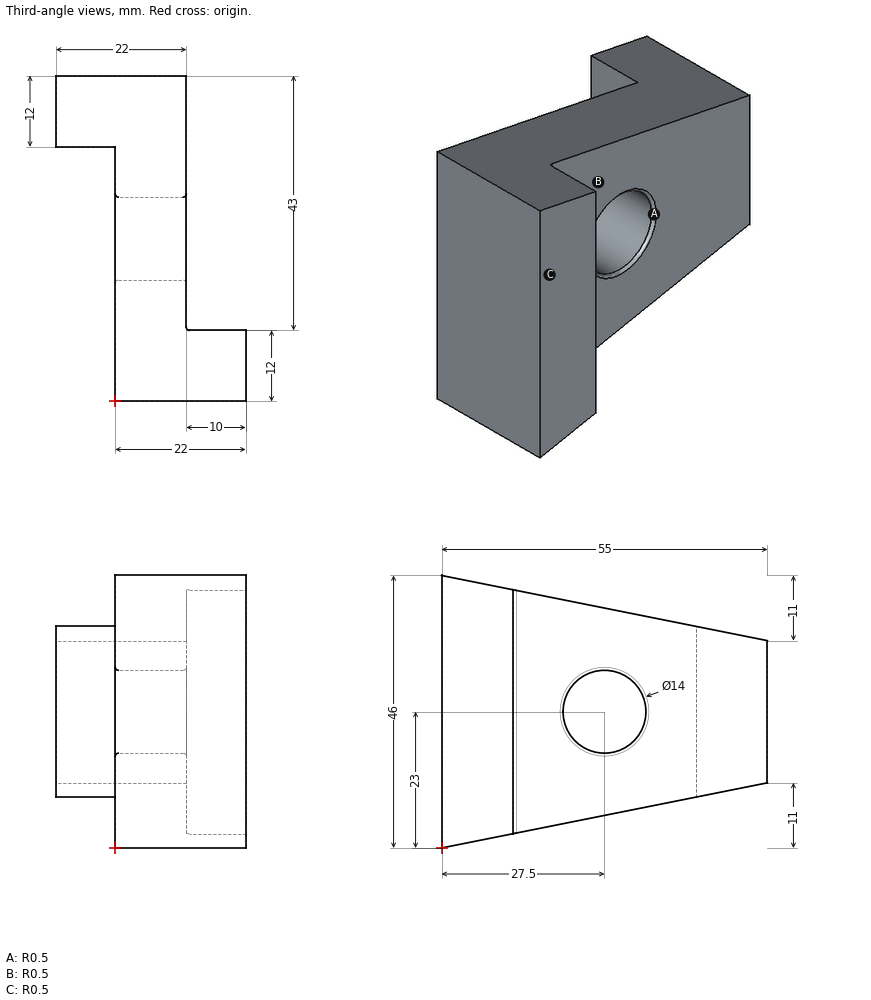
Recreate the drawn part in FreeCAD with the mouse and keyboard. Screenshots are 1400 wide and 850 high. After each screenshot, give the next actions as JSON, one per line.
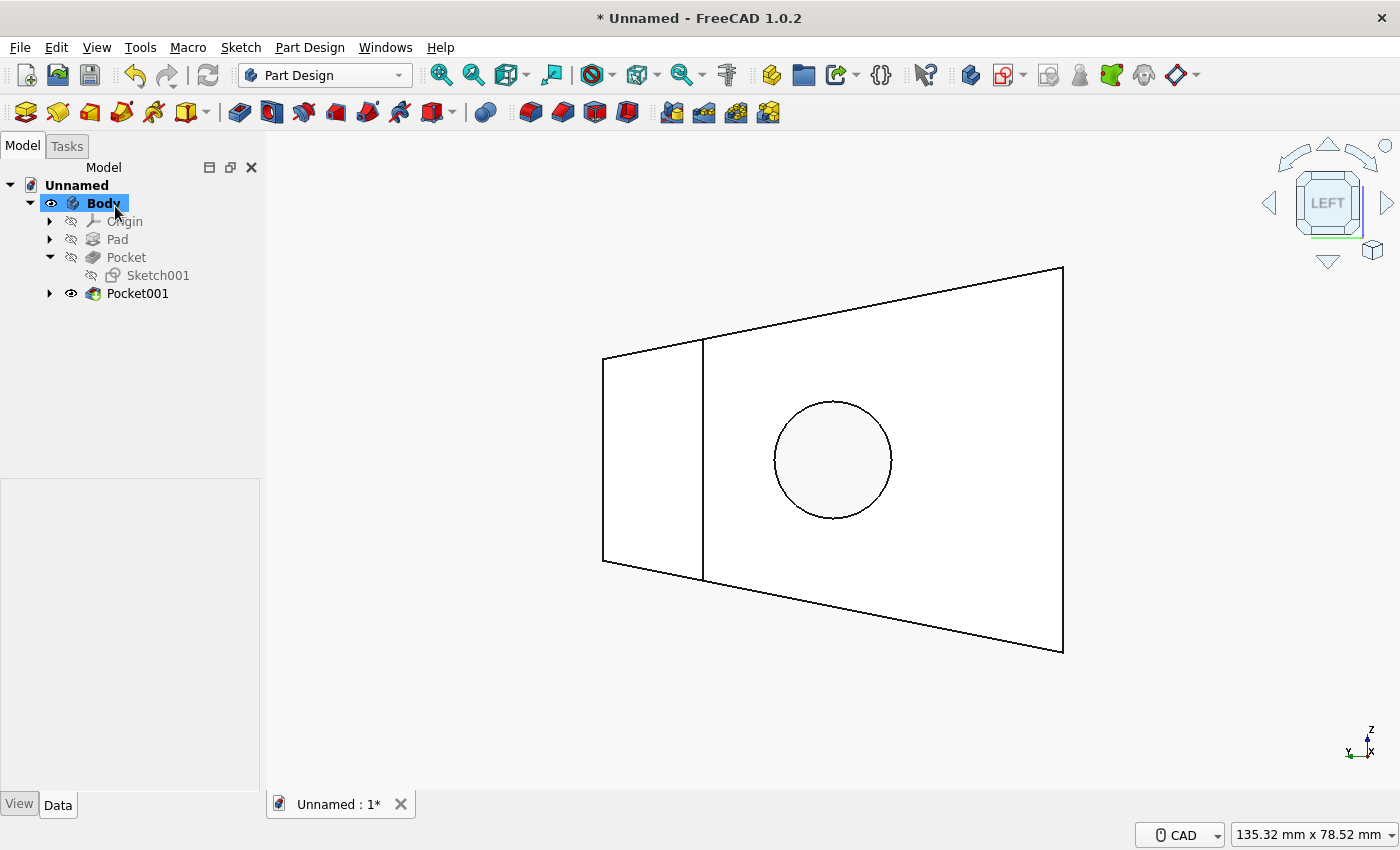
{"action": "key", "text": "0"}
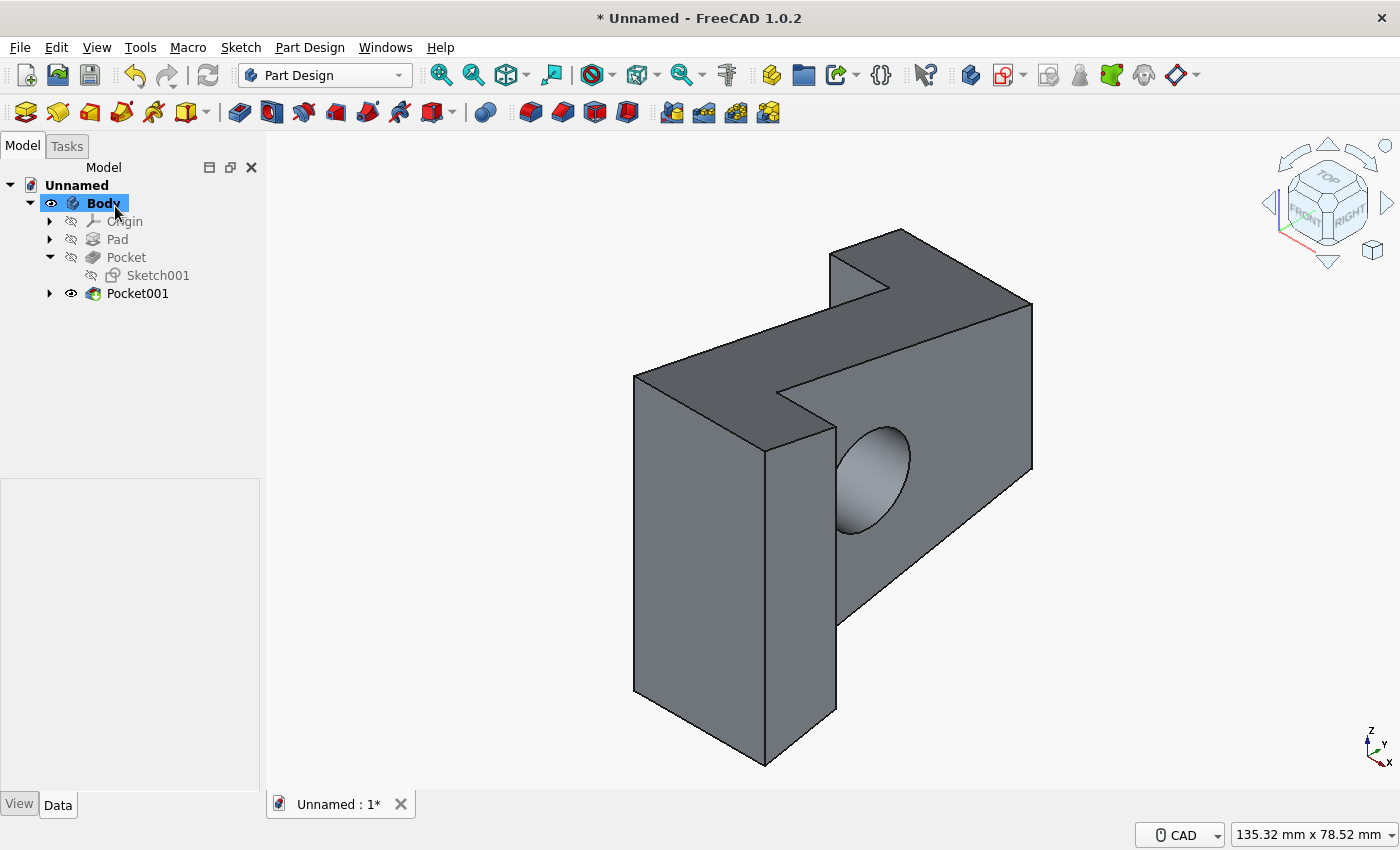
{"action": "left_click", "coordinate": [910, 456]}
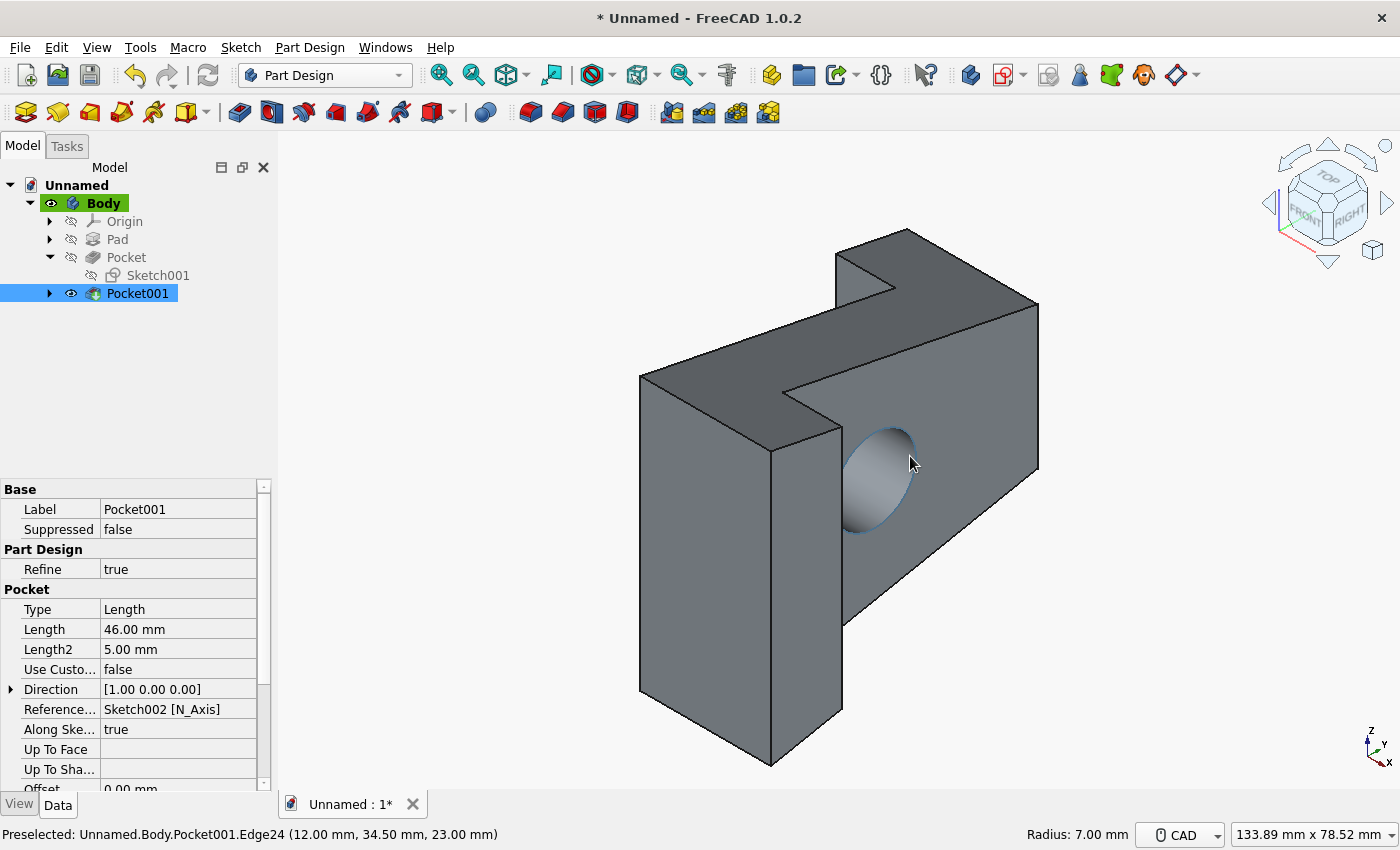
{"action": "left_click", "coordinate": [532, 112]}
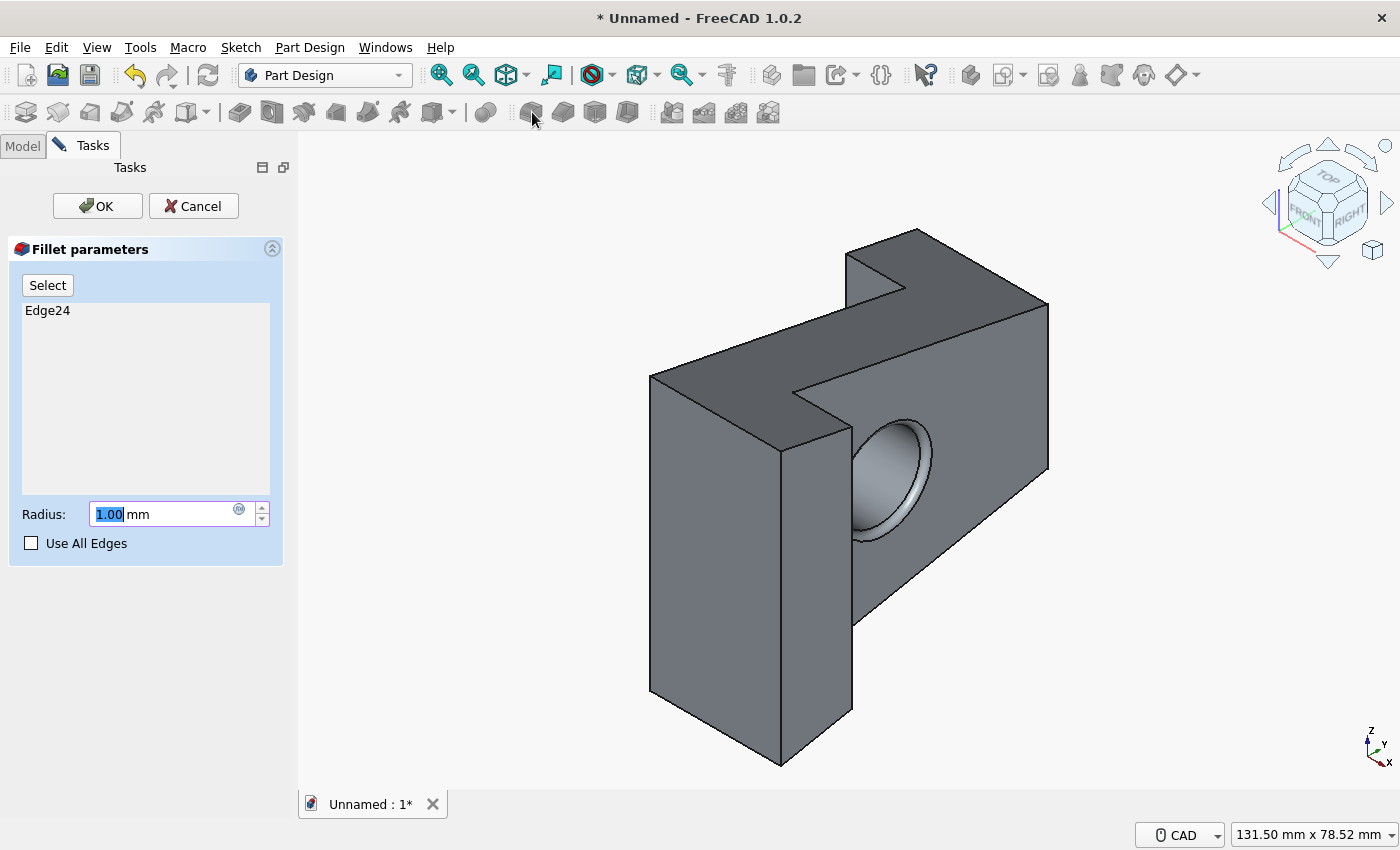
{"action": "type", "text": "0.5"}
{"action": "key", "text": "Tab"}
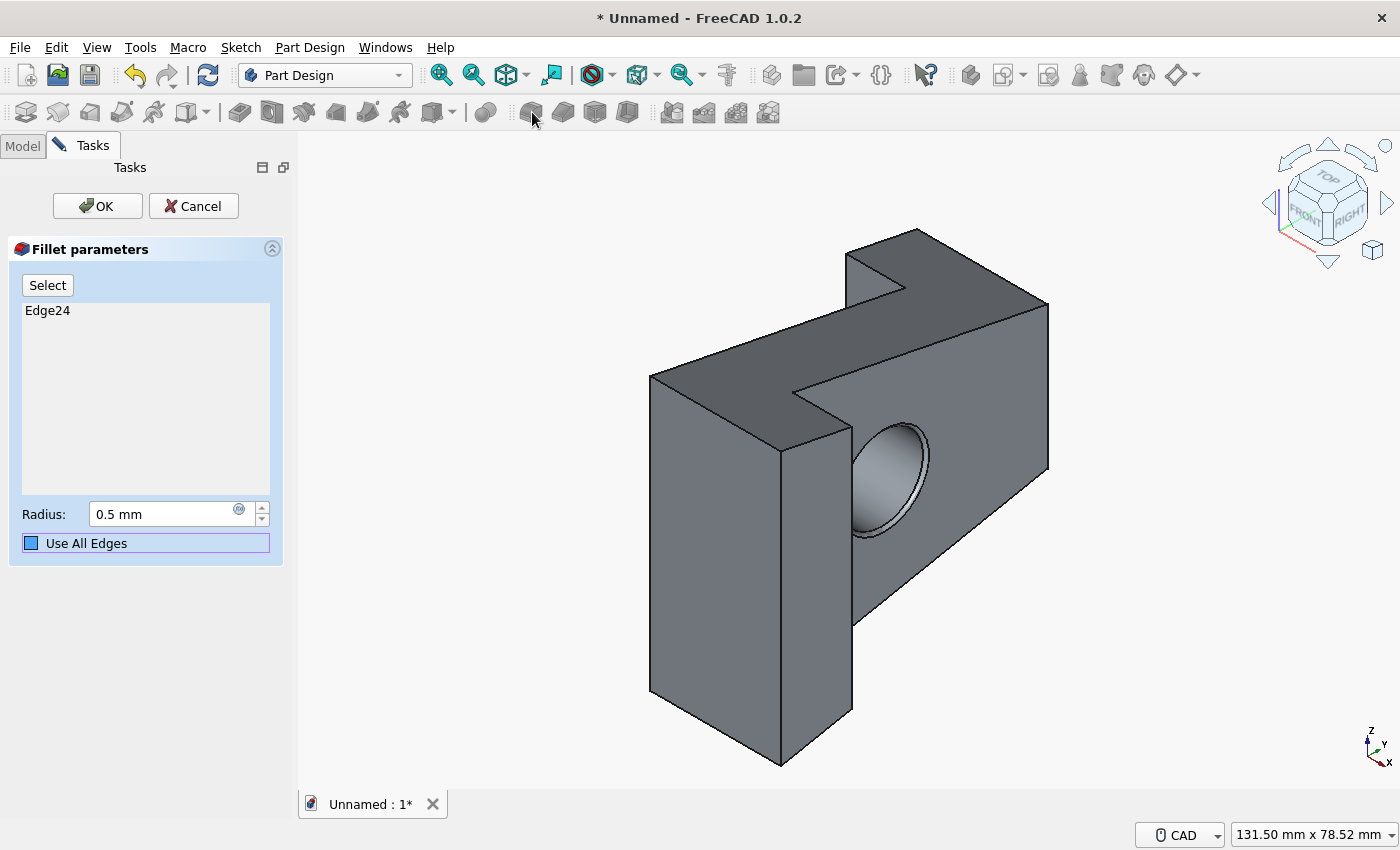
{"action": "left_click", "coordinate": [98, 206]}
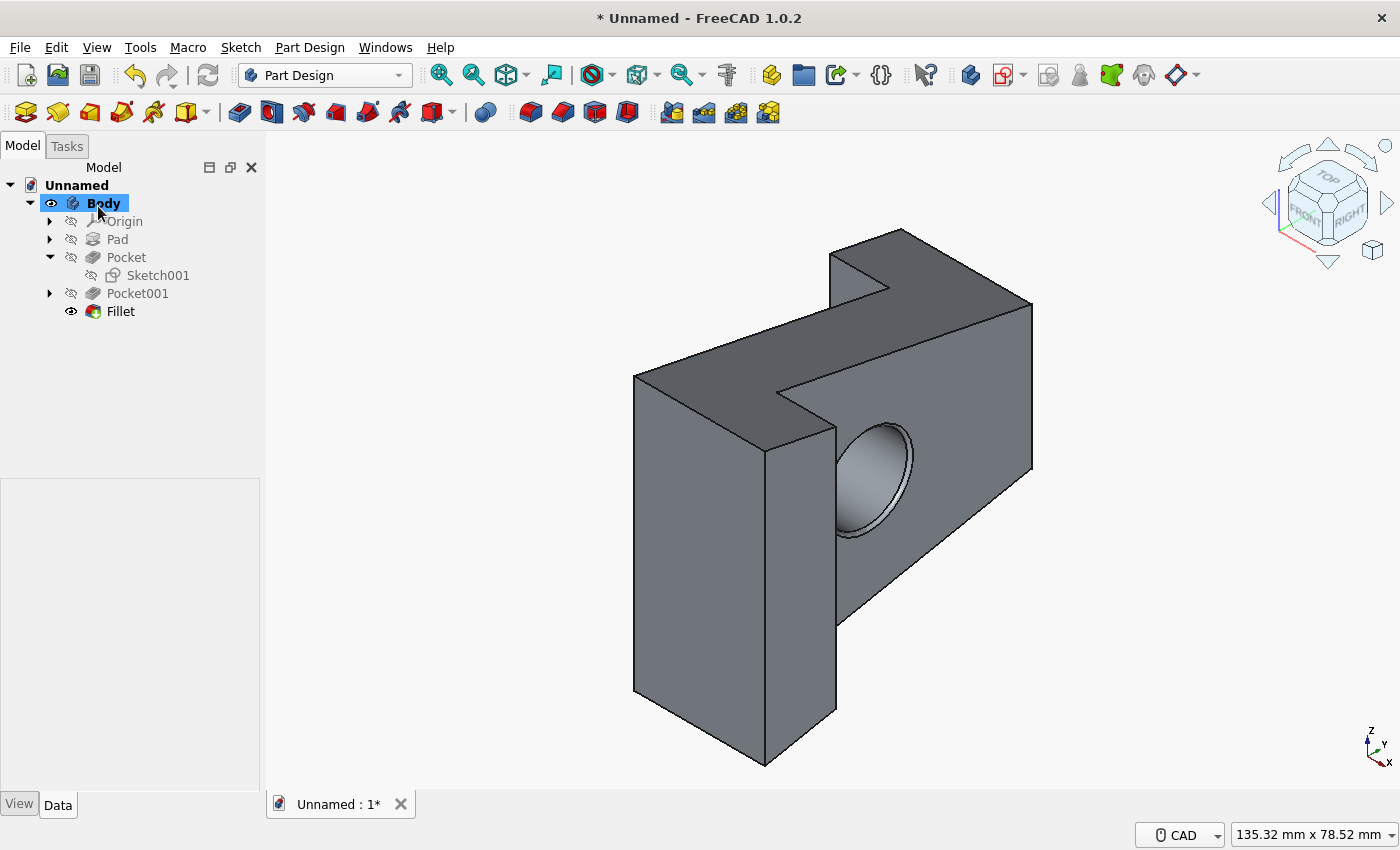
{"action": "key", "text": "2"}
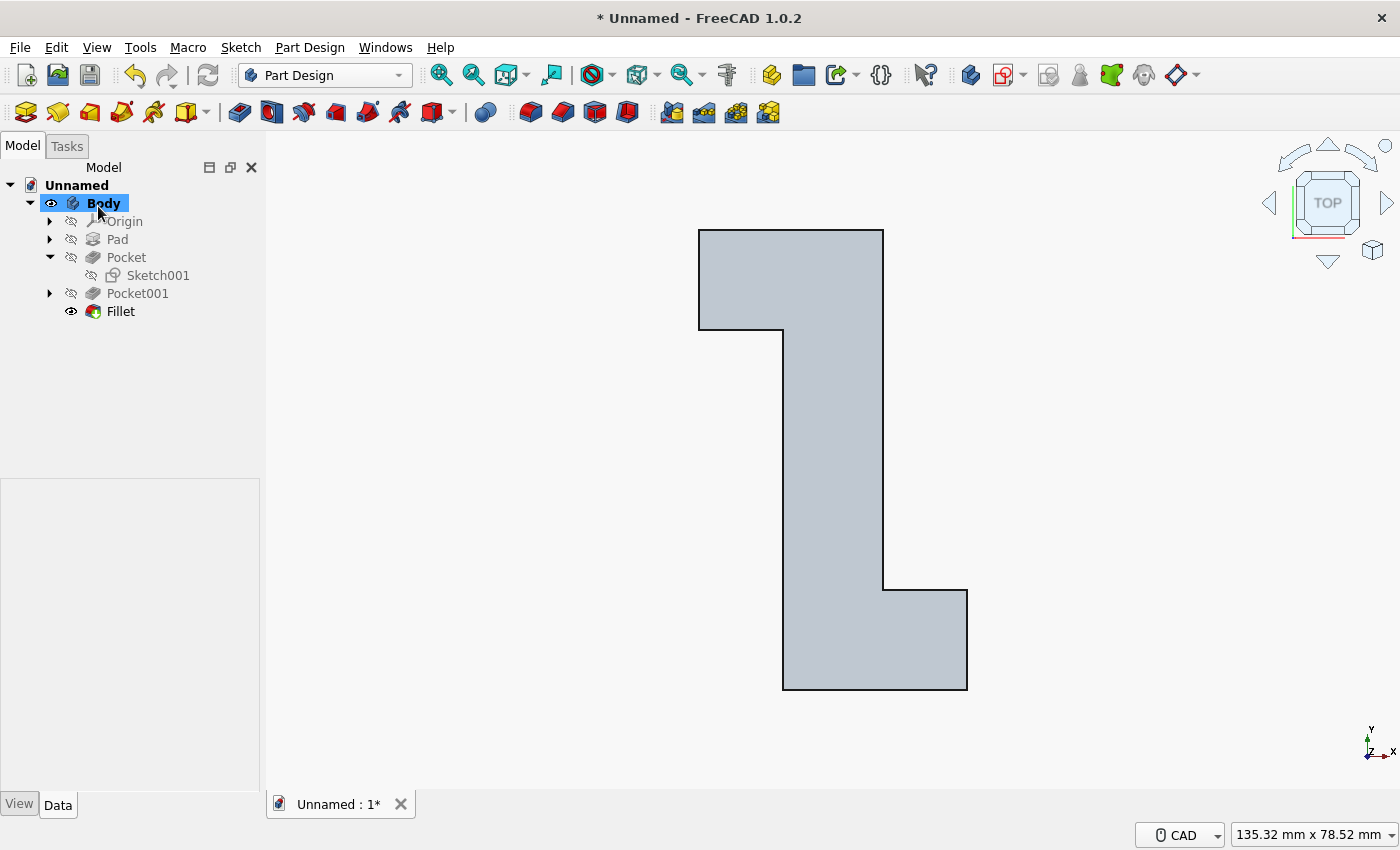
{"action": "key", "text": "0"}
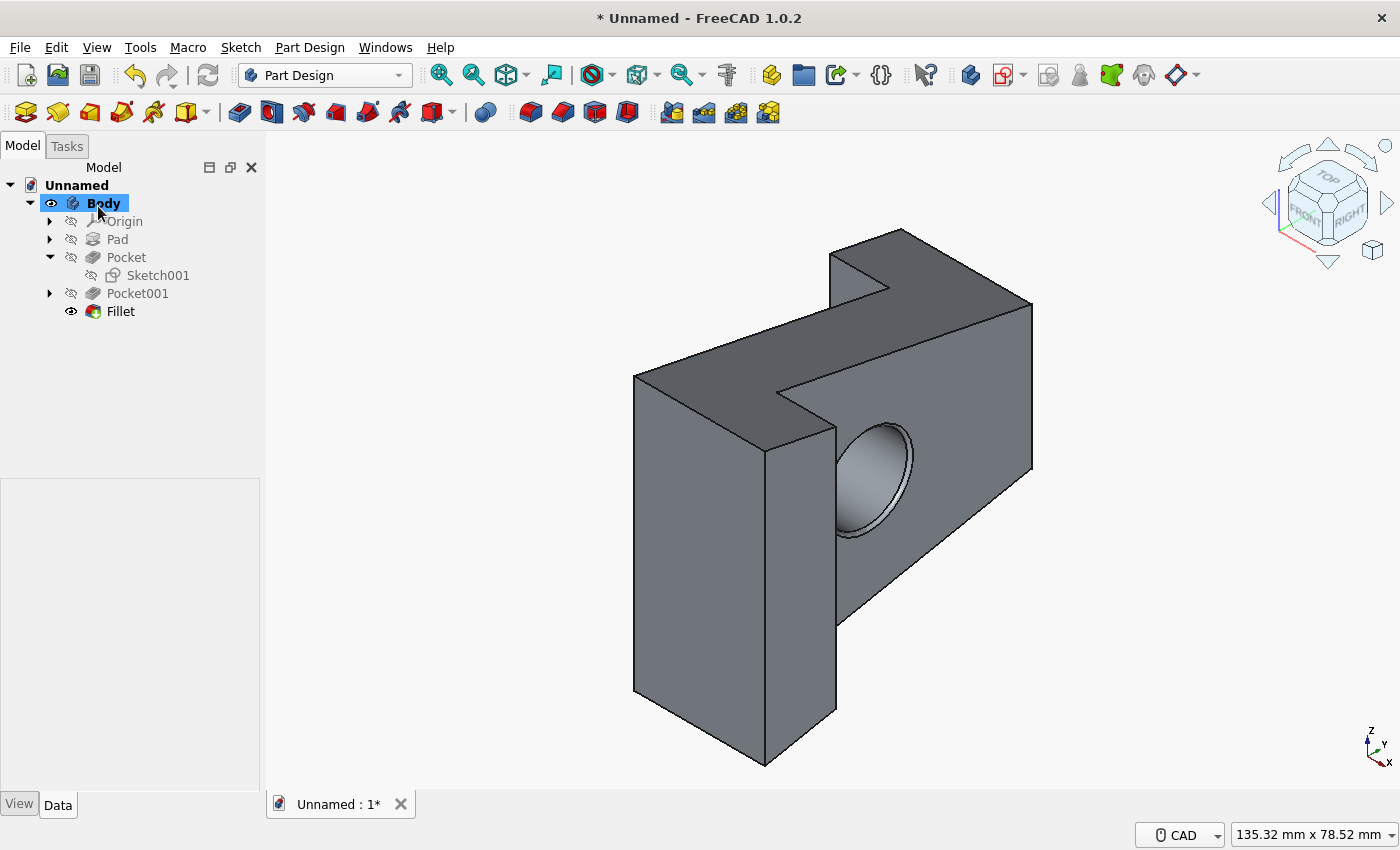
{"action": "key", "text": "1"}